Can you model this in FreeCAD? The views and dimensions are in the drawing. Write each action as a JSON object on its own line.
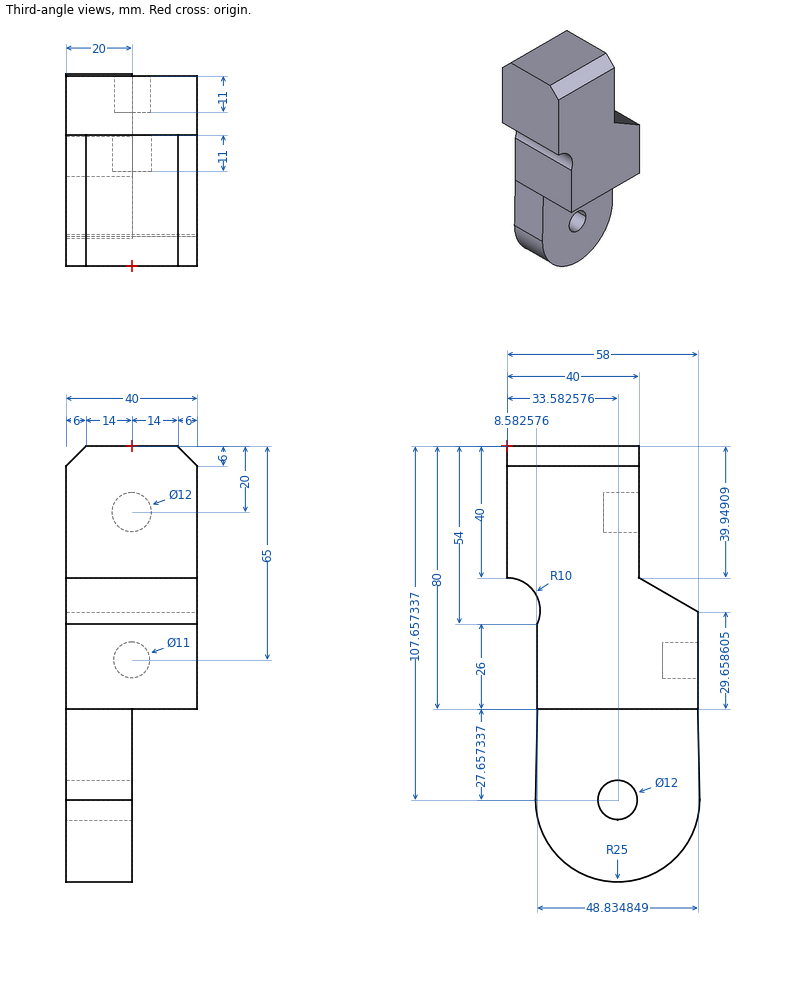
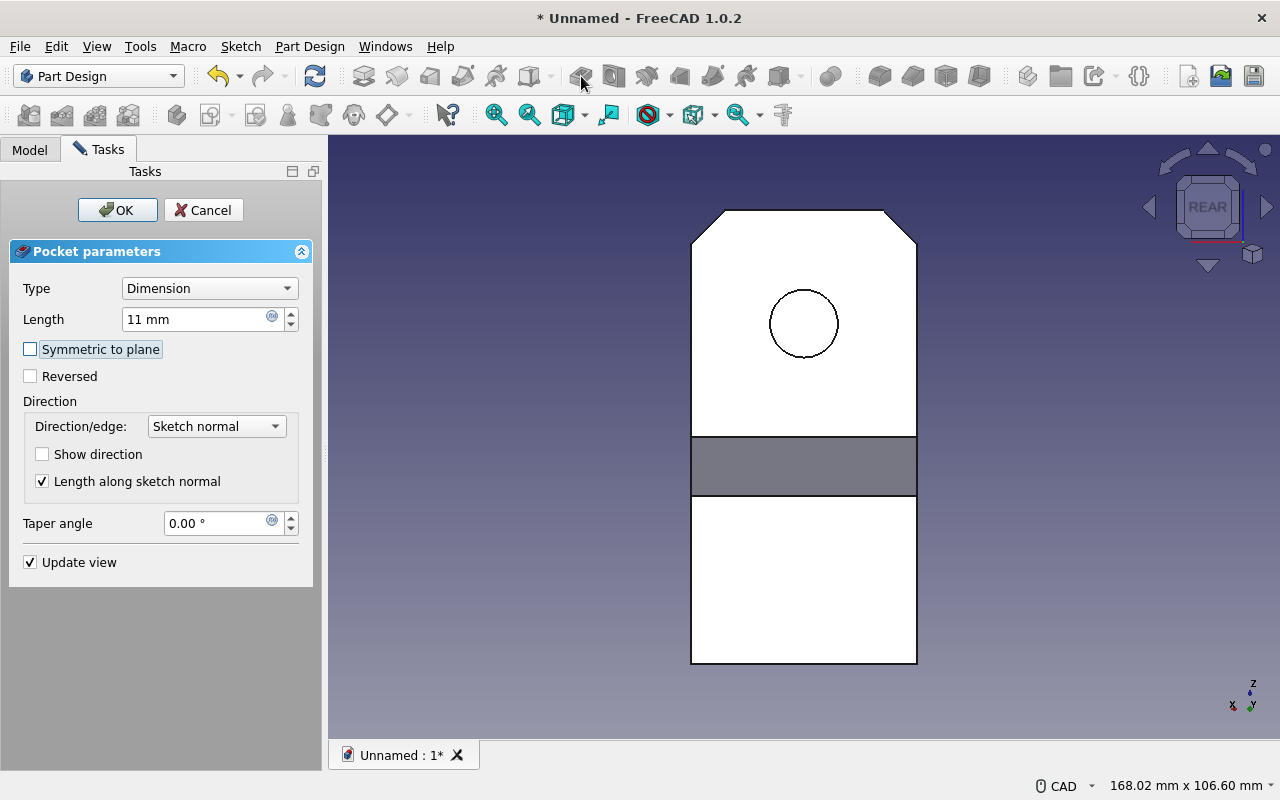
{"action": "left_click", "coordinate": [118, 210]}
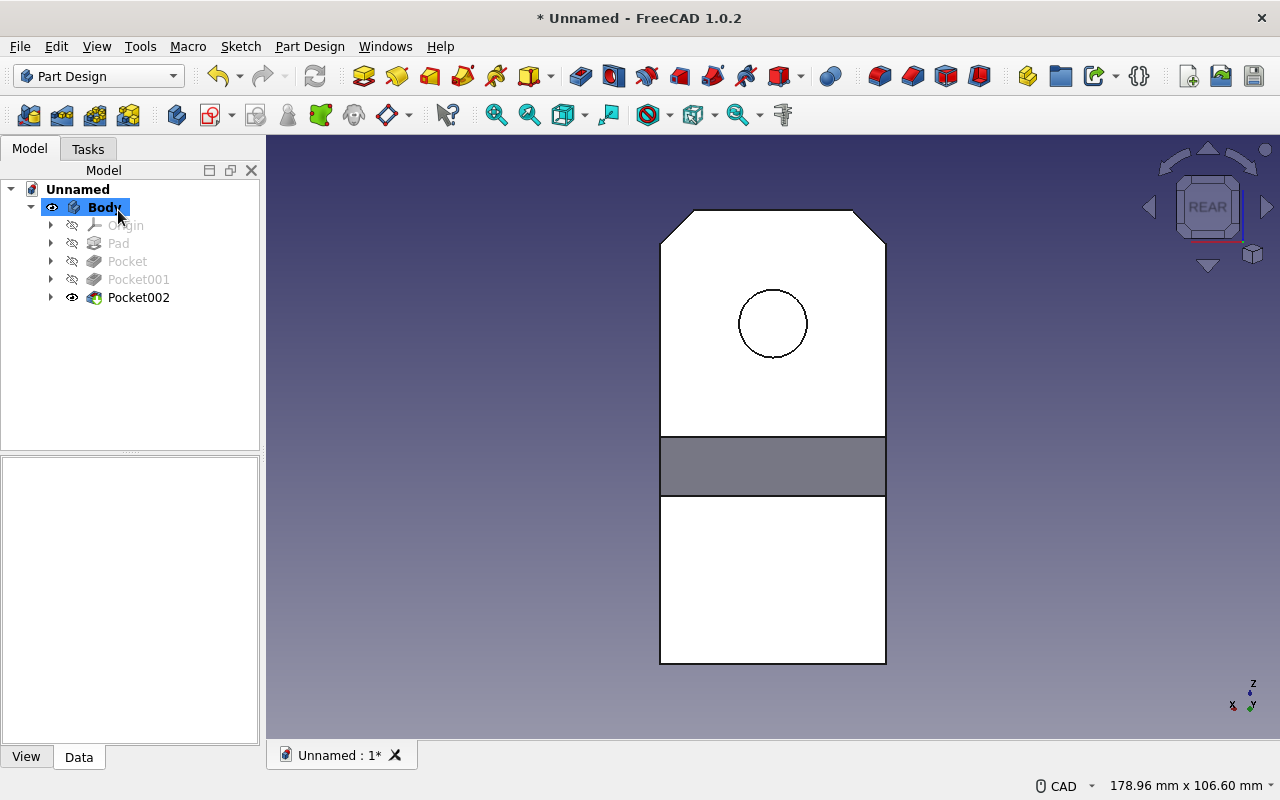
{"action": "left_click", "coordinate": [773, 579]}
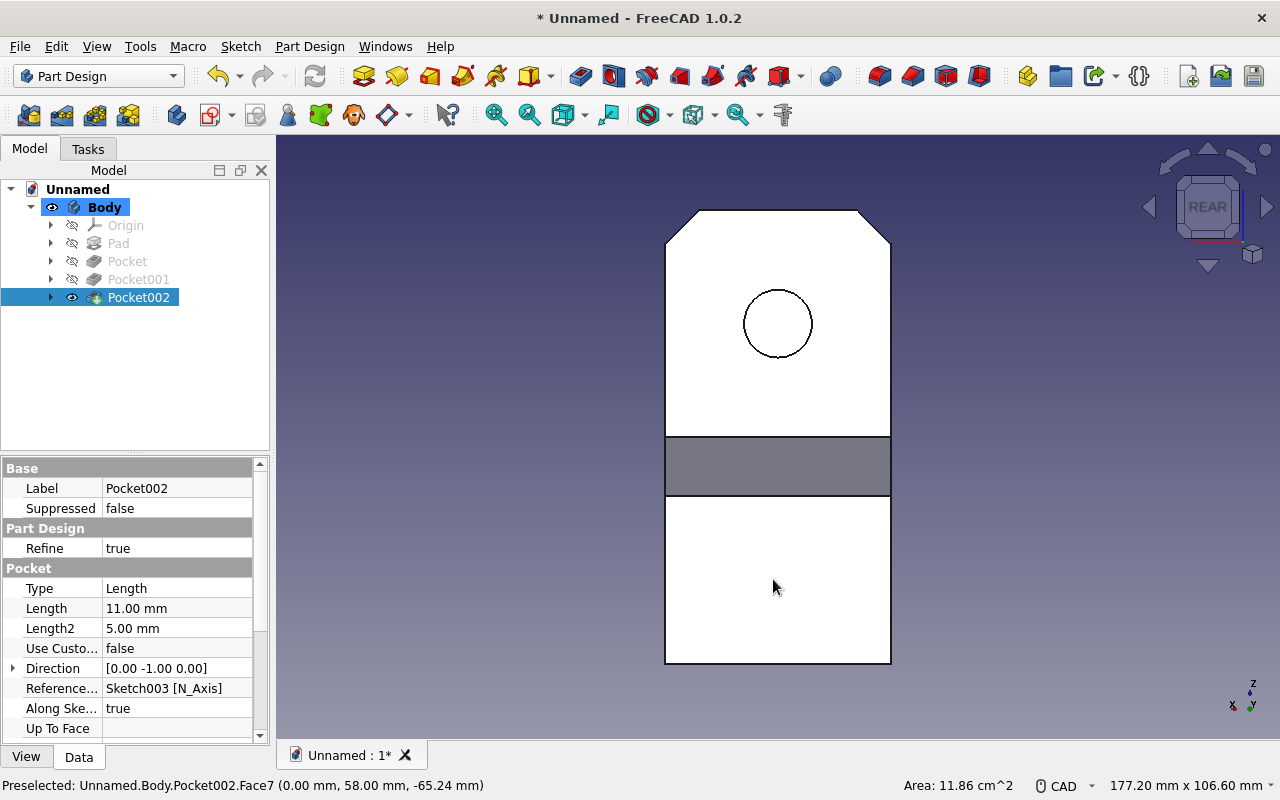
{"action": "left_click", "coordinate": [210, 116]}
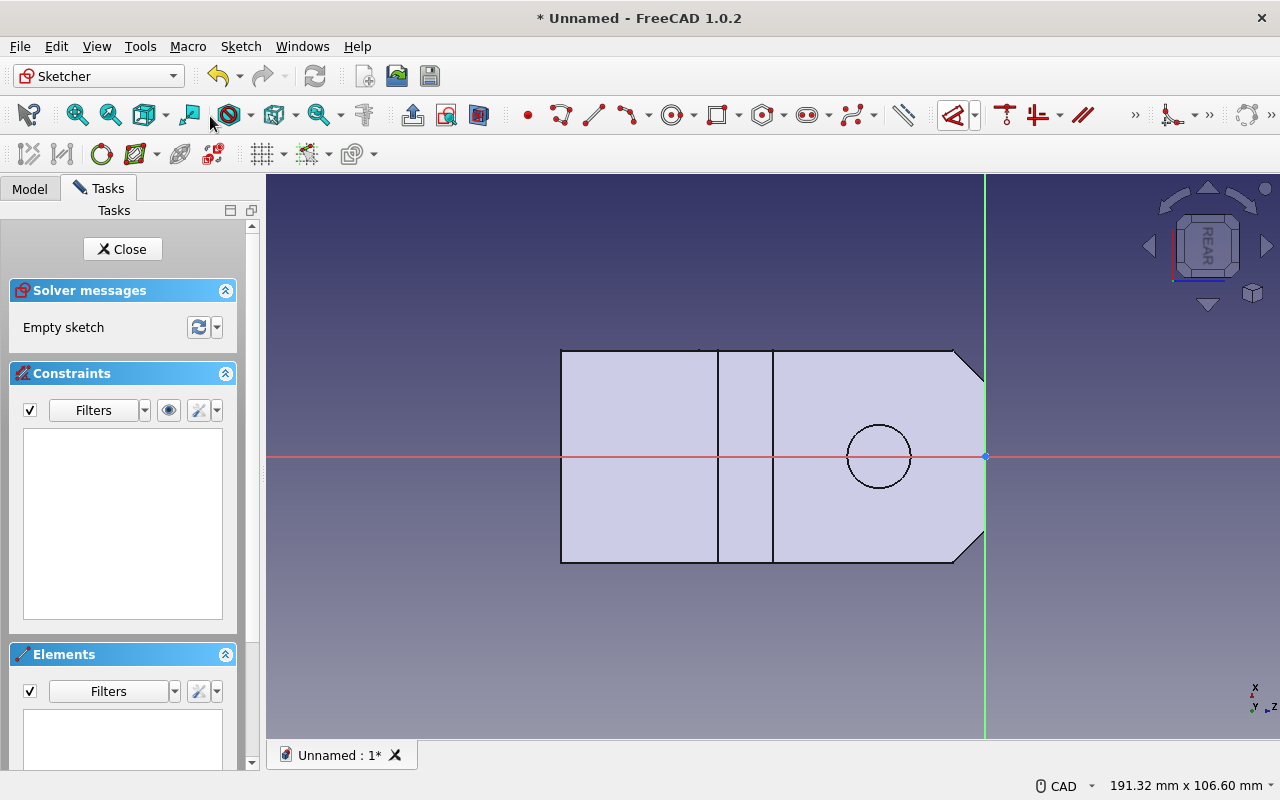
{"action": "scroll", "coordinate": [628, 457], "scroll_direction": "up", "scroll_amount": 9}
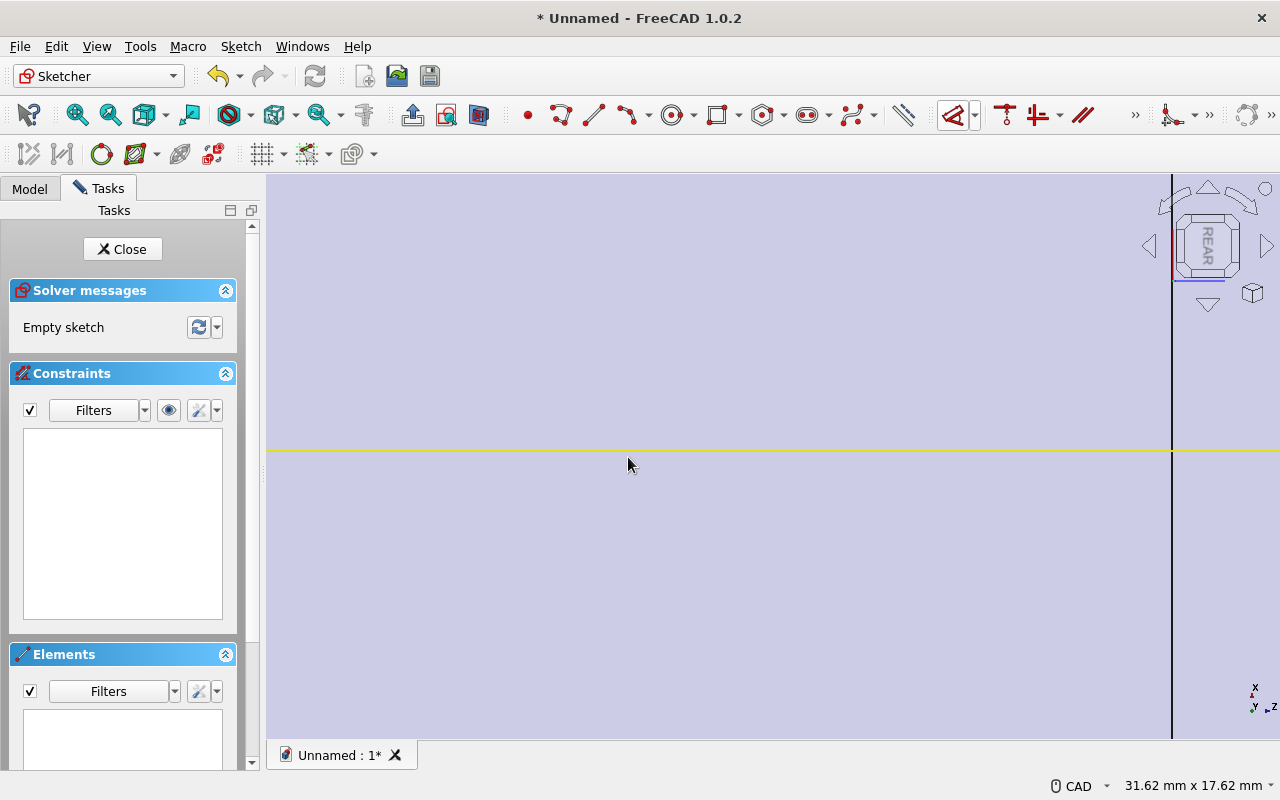
{"action": "key", "text": "g c"}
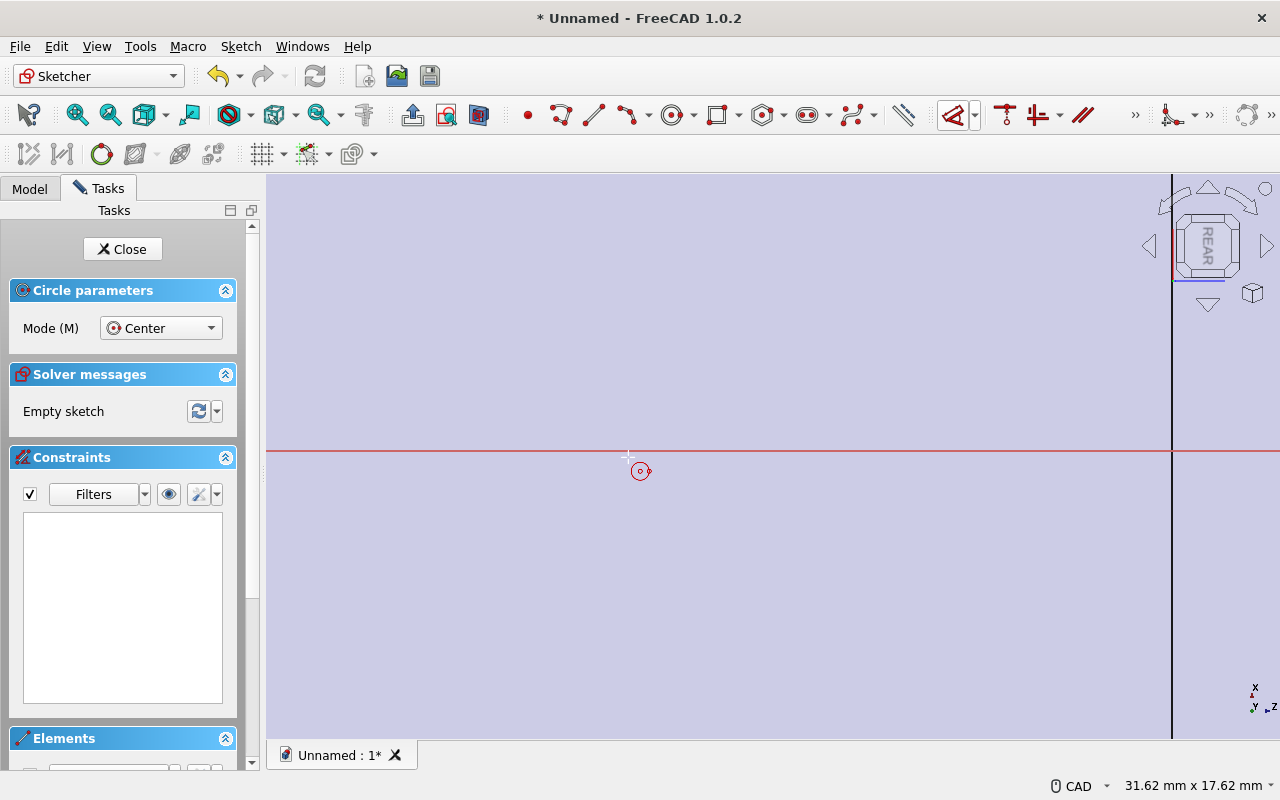
{"action": "left_click", "coordinate": [702, 451]}
{"action": "mouse_move", "coordinate": [827, 327]}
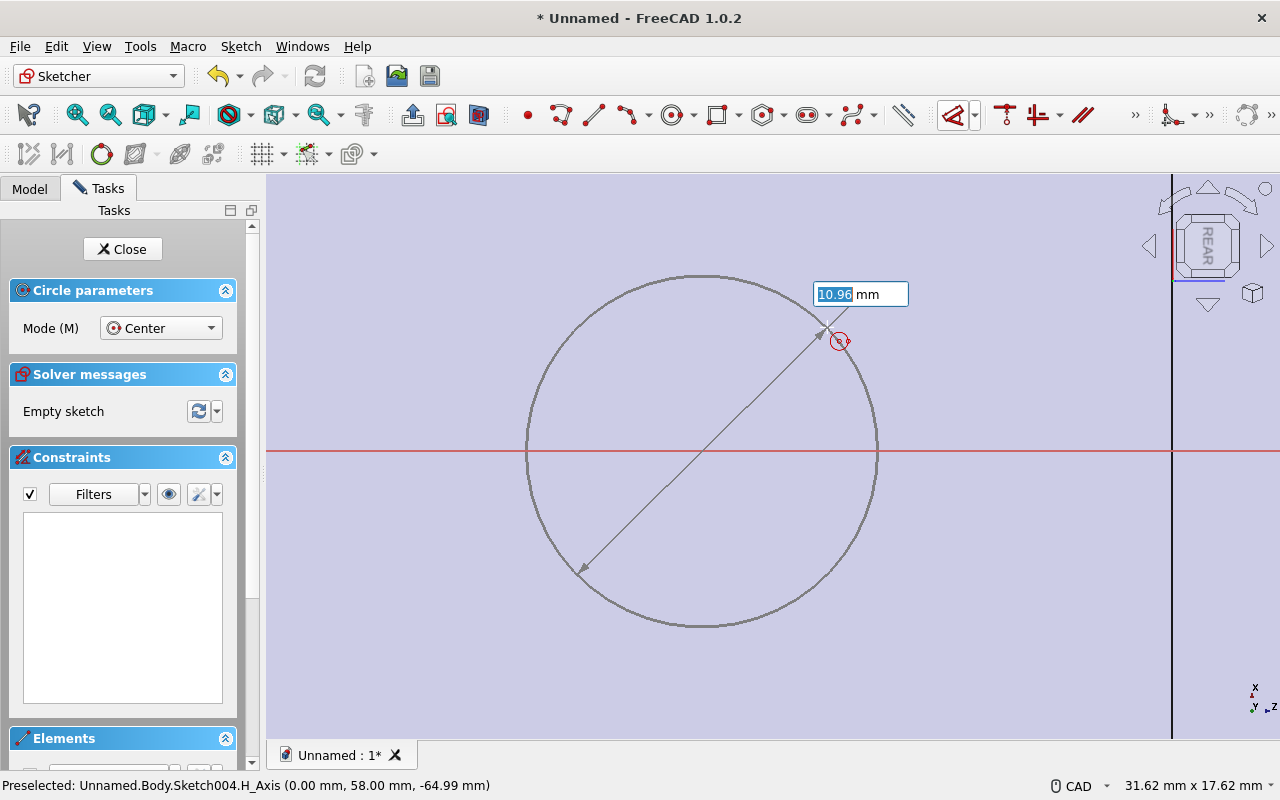
{"action": "type", "text": "11"}
{"action": "key", "text": "Return"}
{"action": "key", "text": "Escape"}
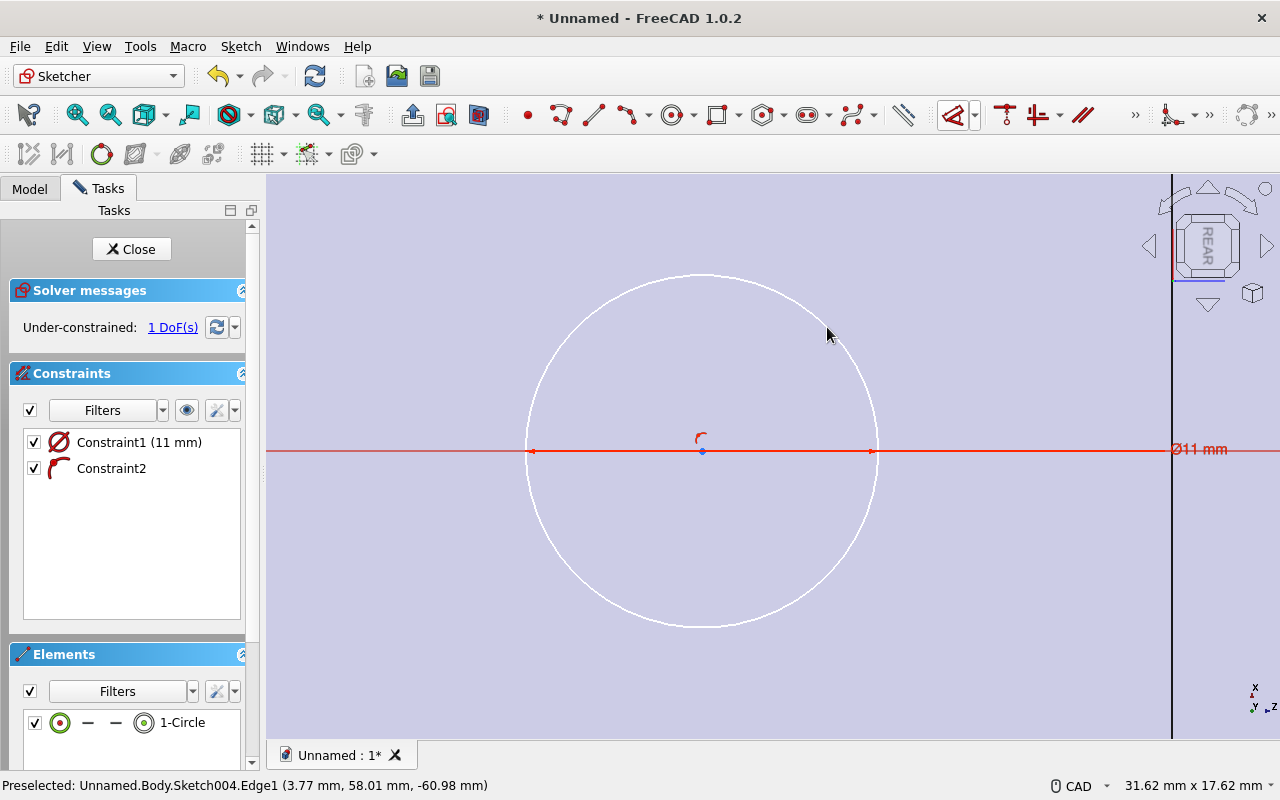
{"action": "left_click", "coordinate": [702, 451]}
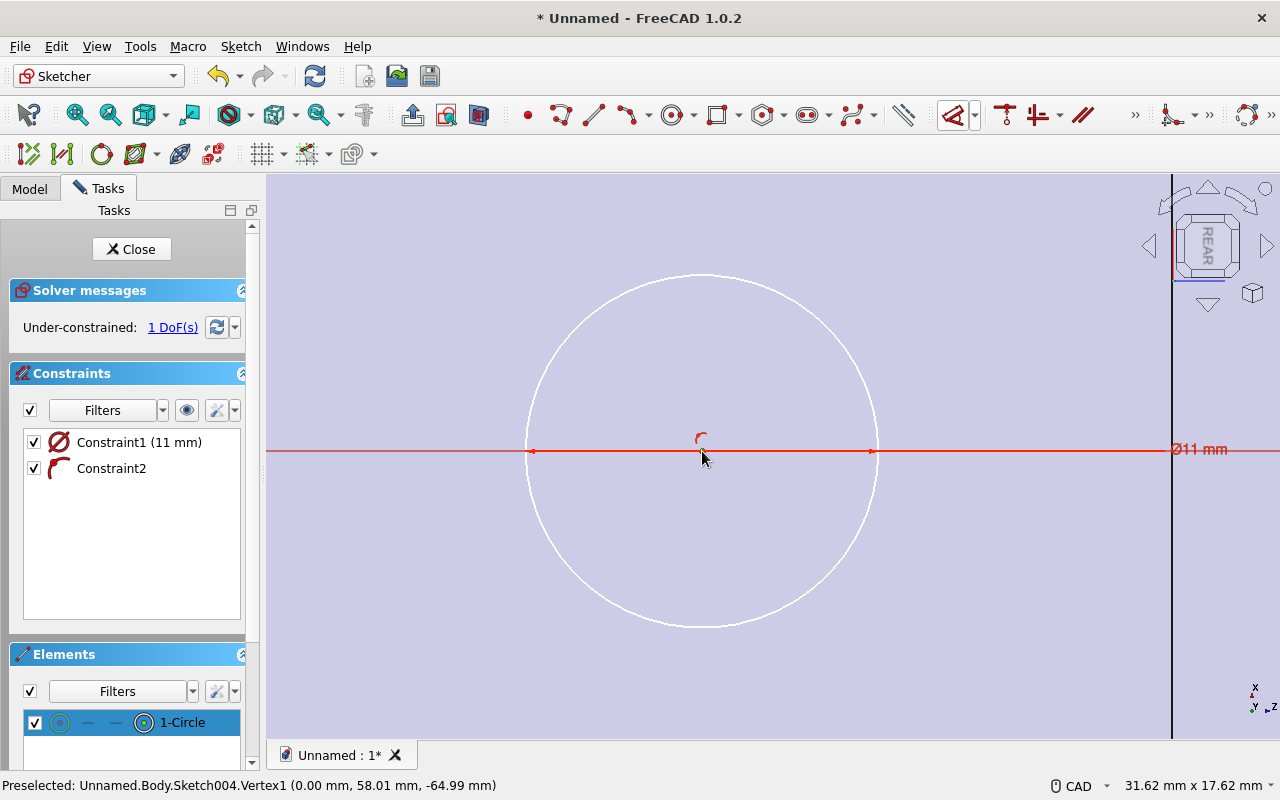
{"action": "key", "text": "l"}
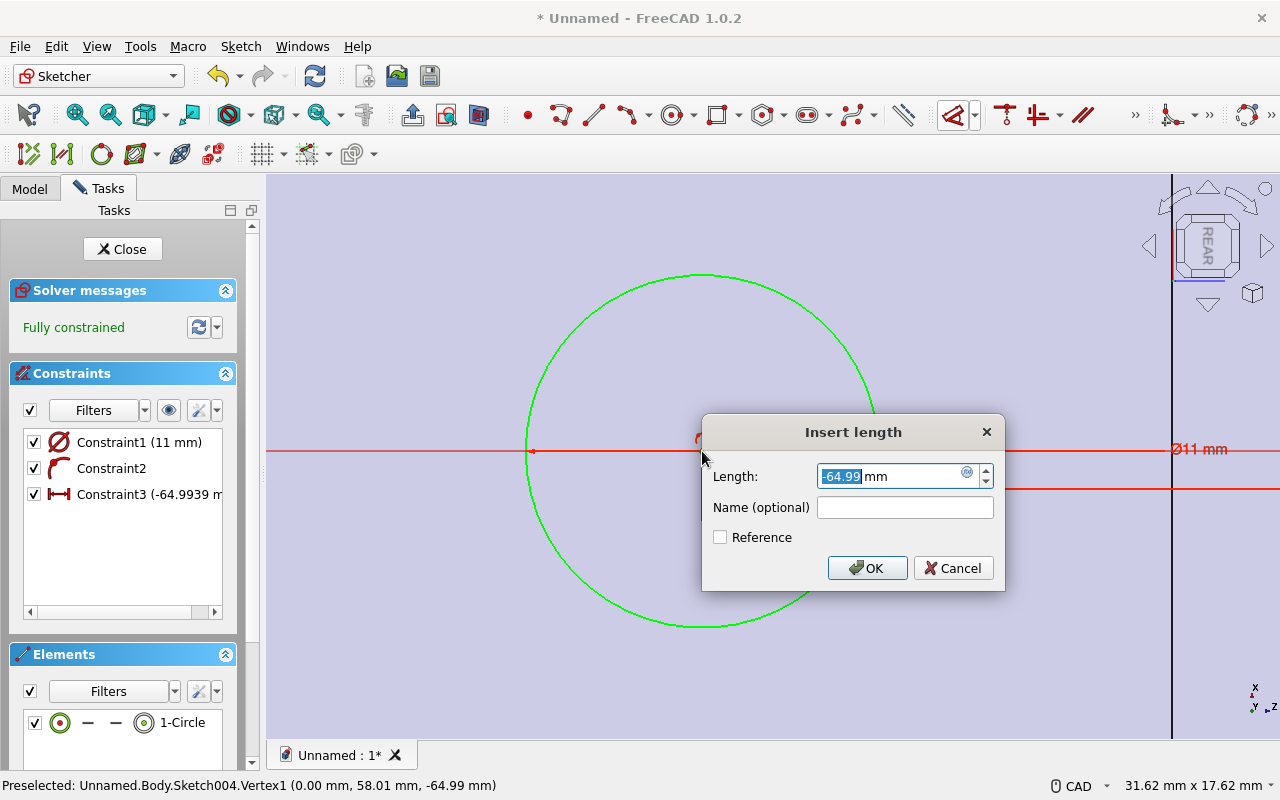
{"action": "type", "text": "-65"}
{"action": "key", "text": "Return"}